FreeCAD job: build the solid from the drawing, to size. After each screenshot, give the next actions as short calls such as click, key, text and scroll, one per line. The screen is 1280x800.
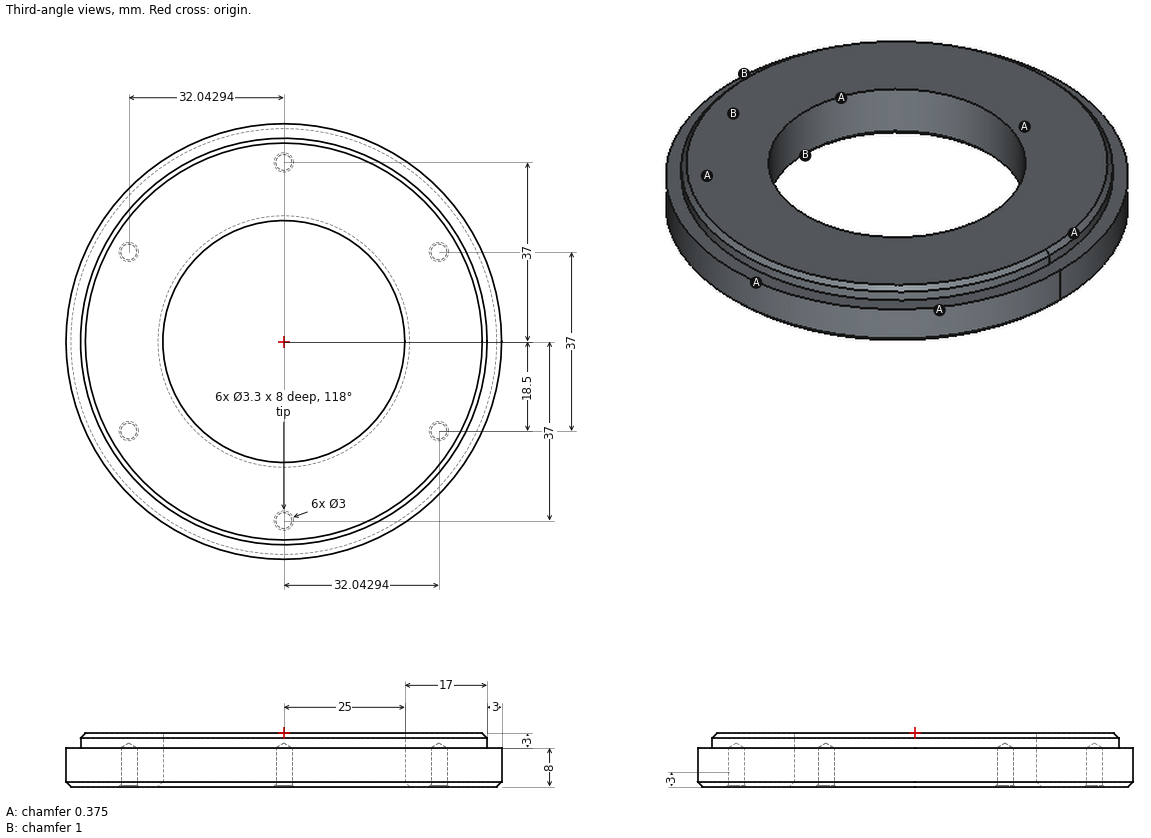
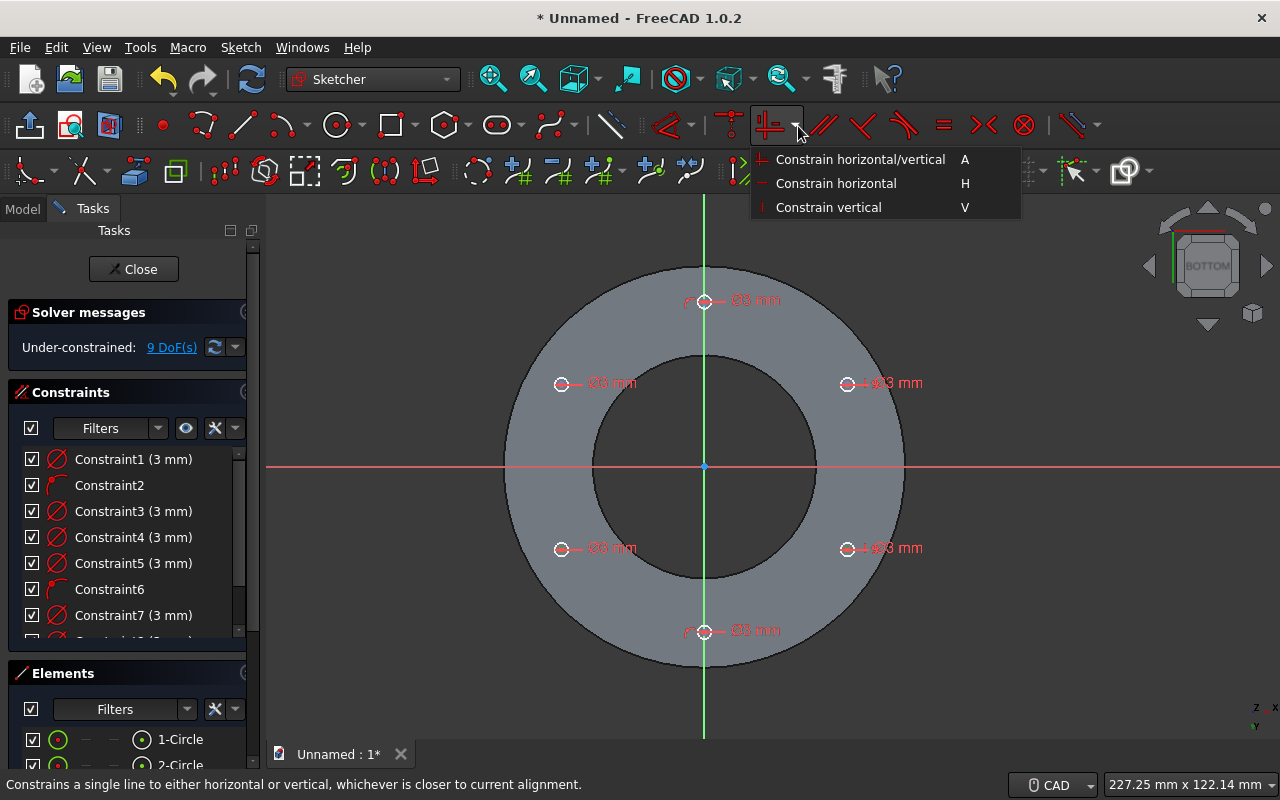
click(886, 183)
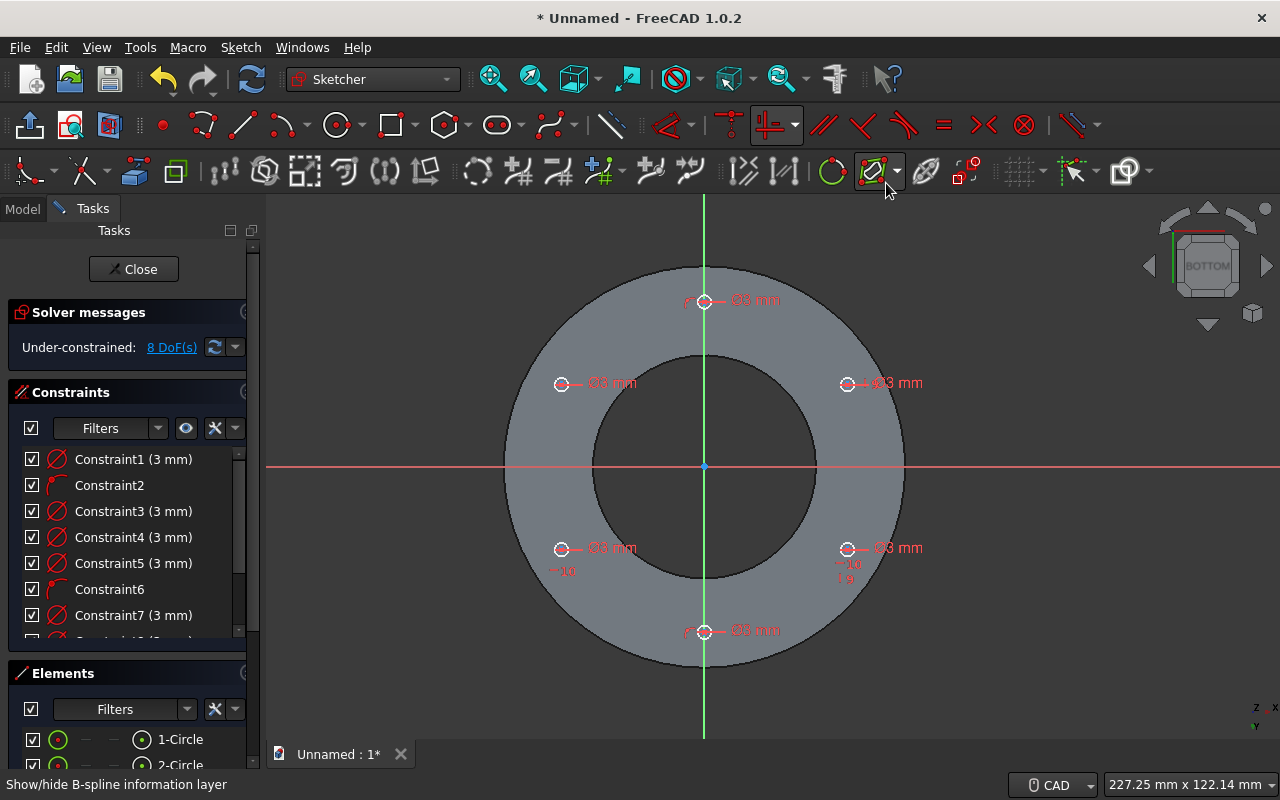
click(561, 550)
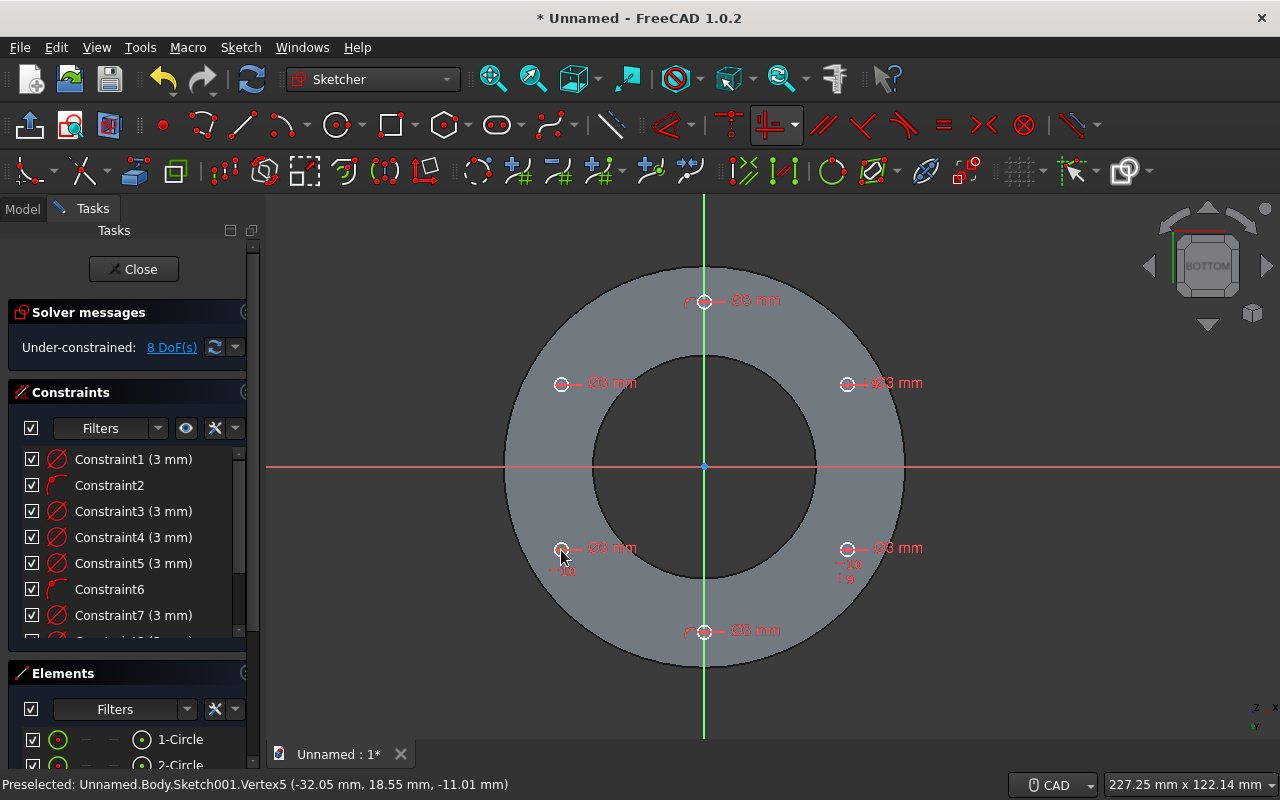
click(561, 385)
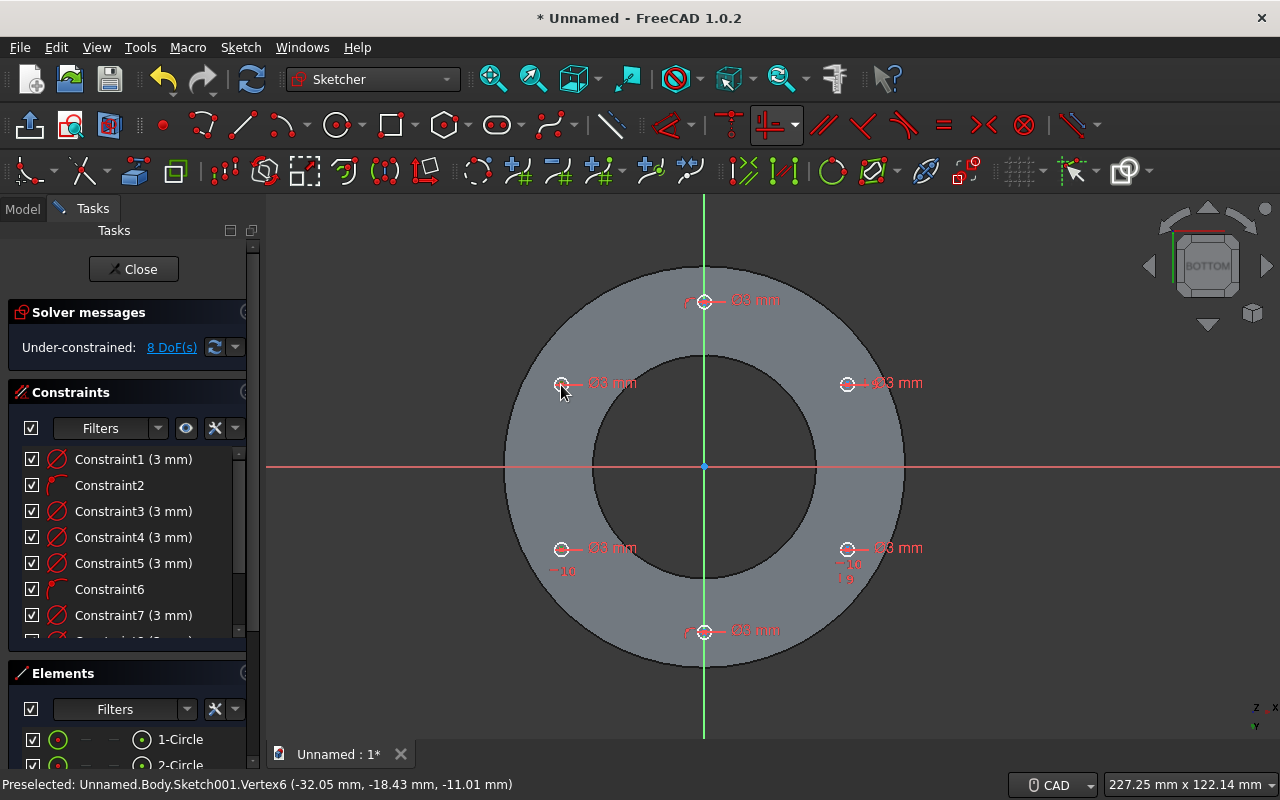
click(798, 126)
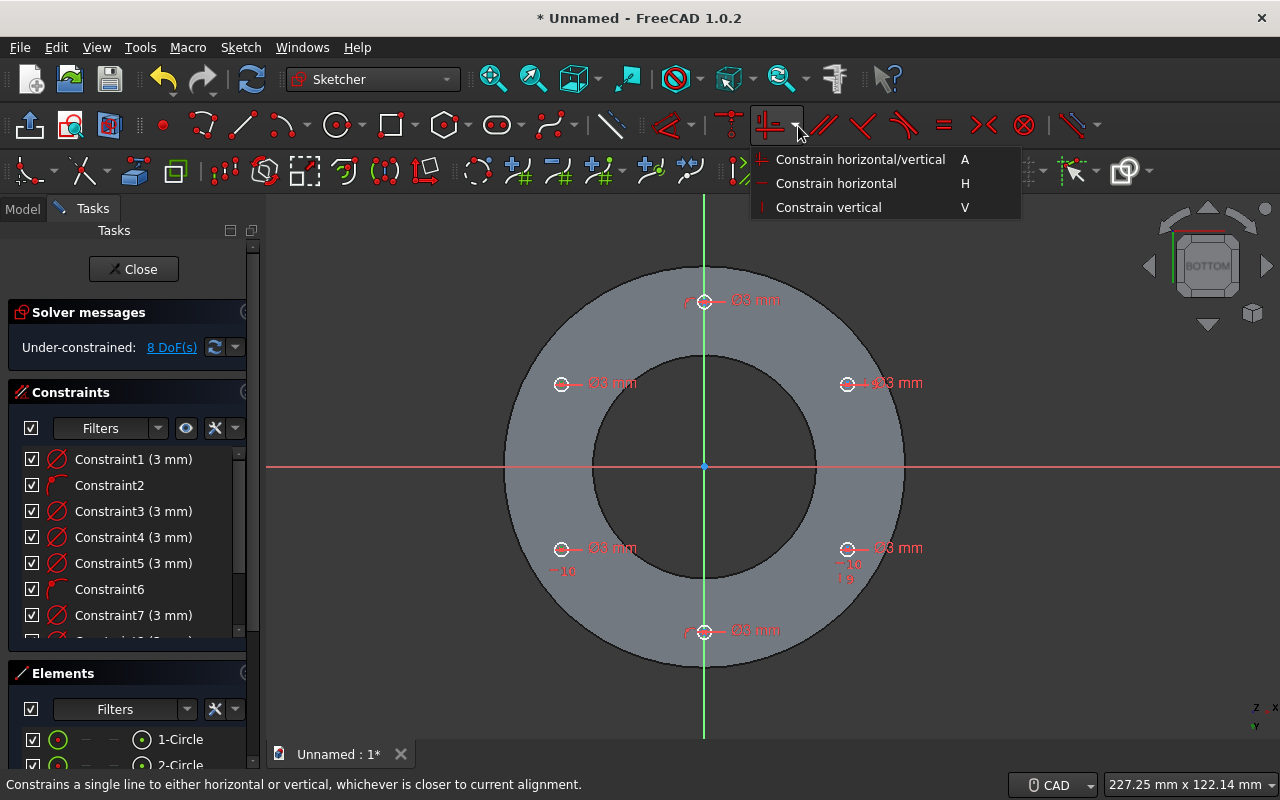
click(886, 207)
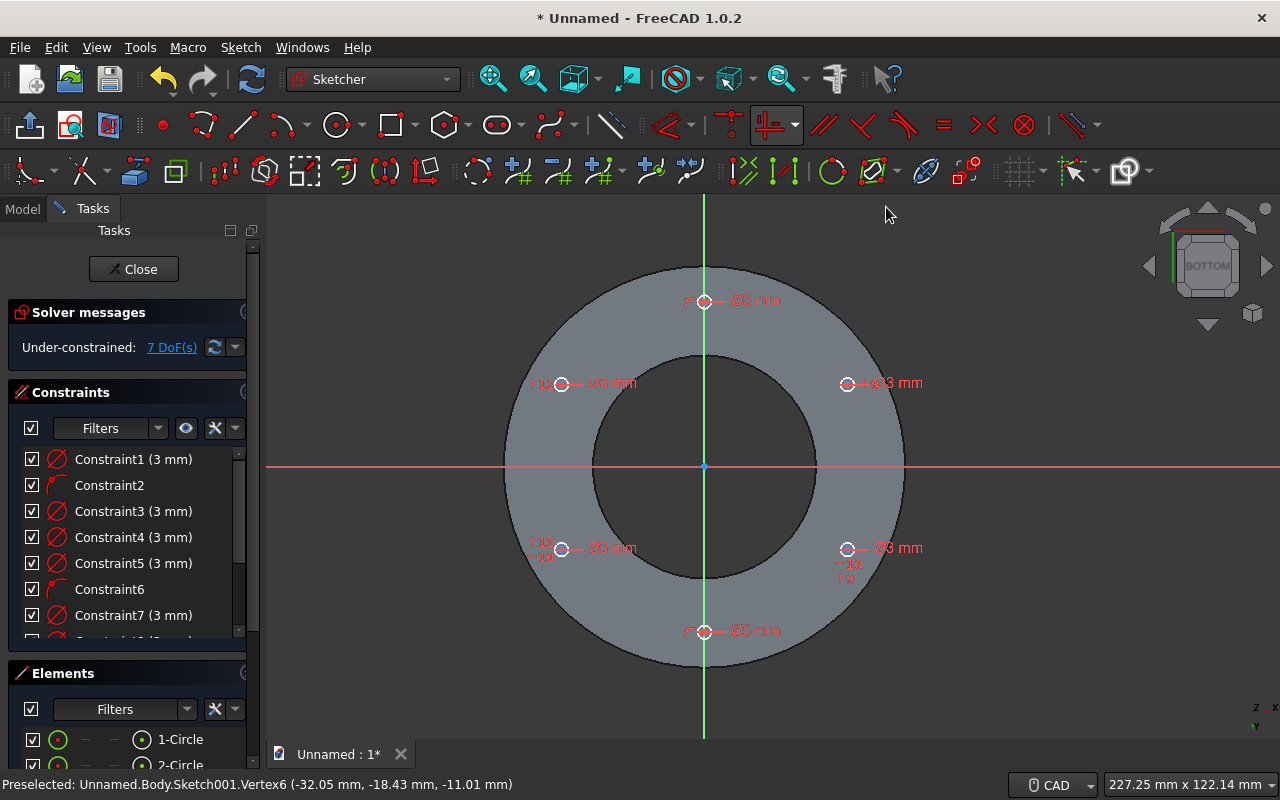
click(847, 385)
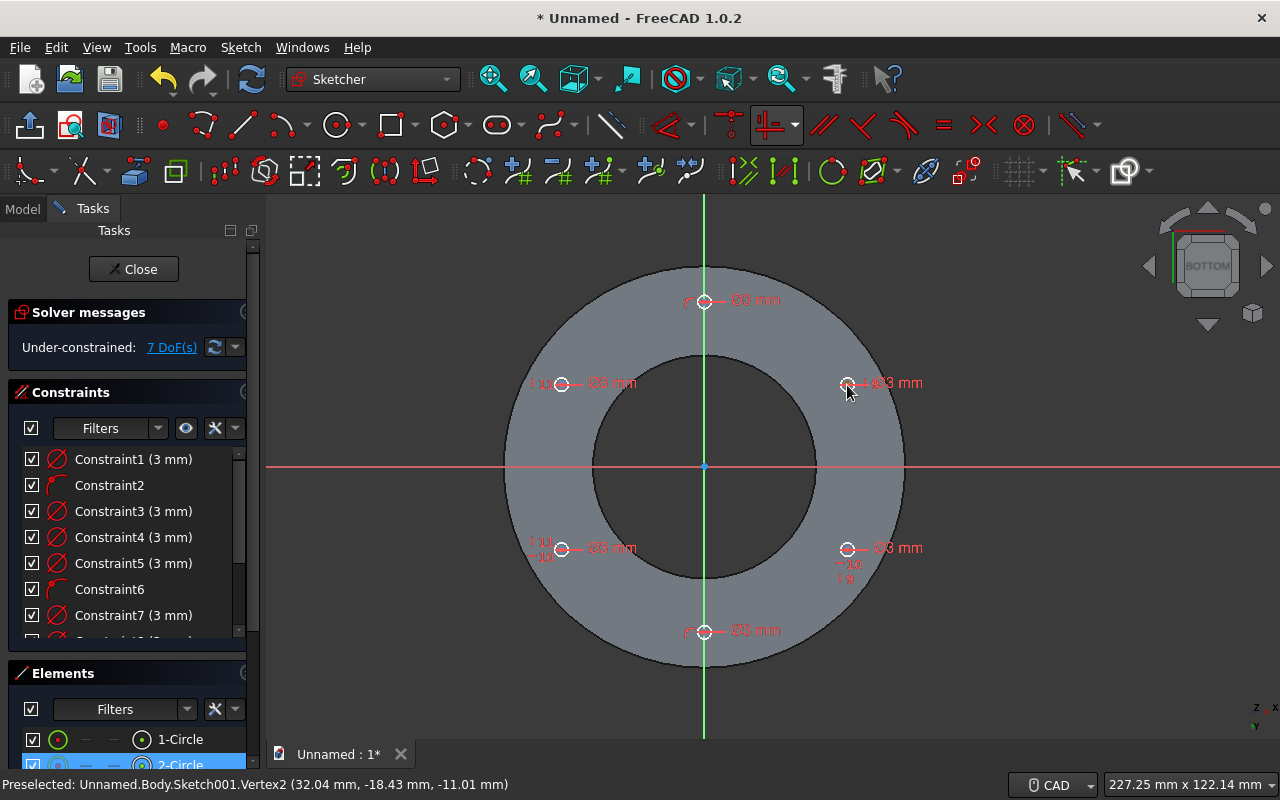
click(561, 385)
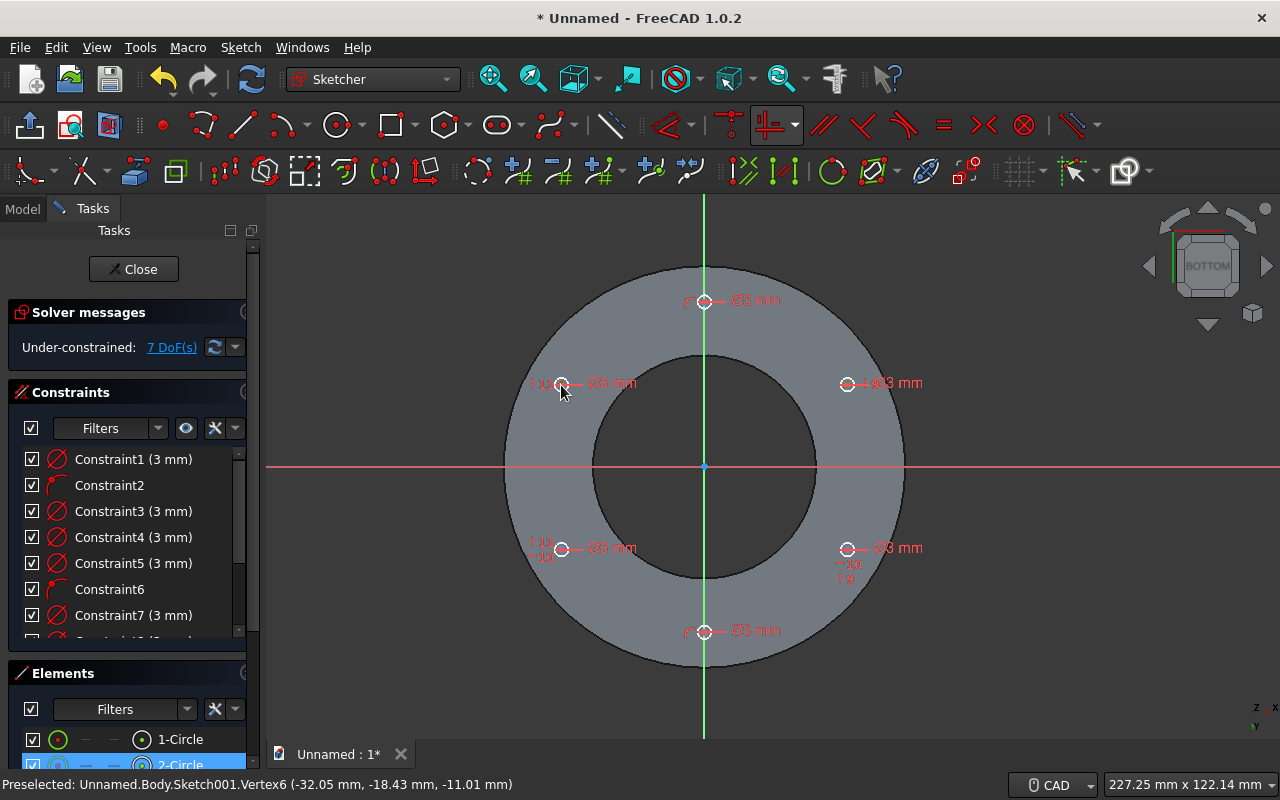
click(798, 126)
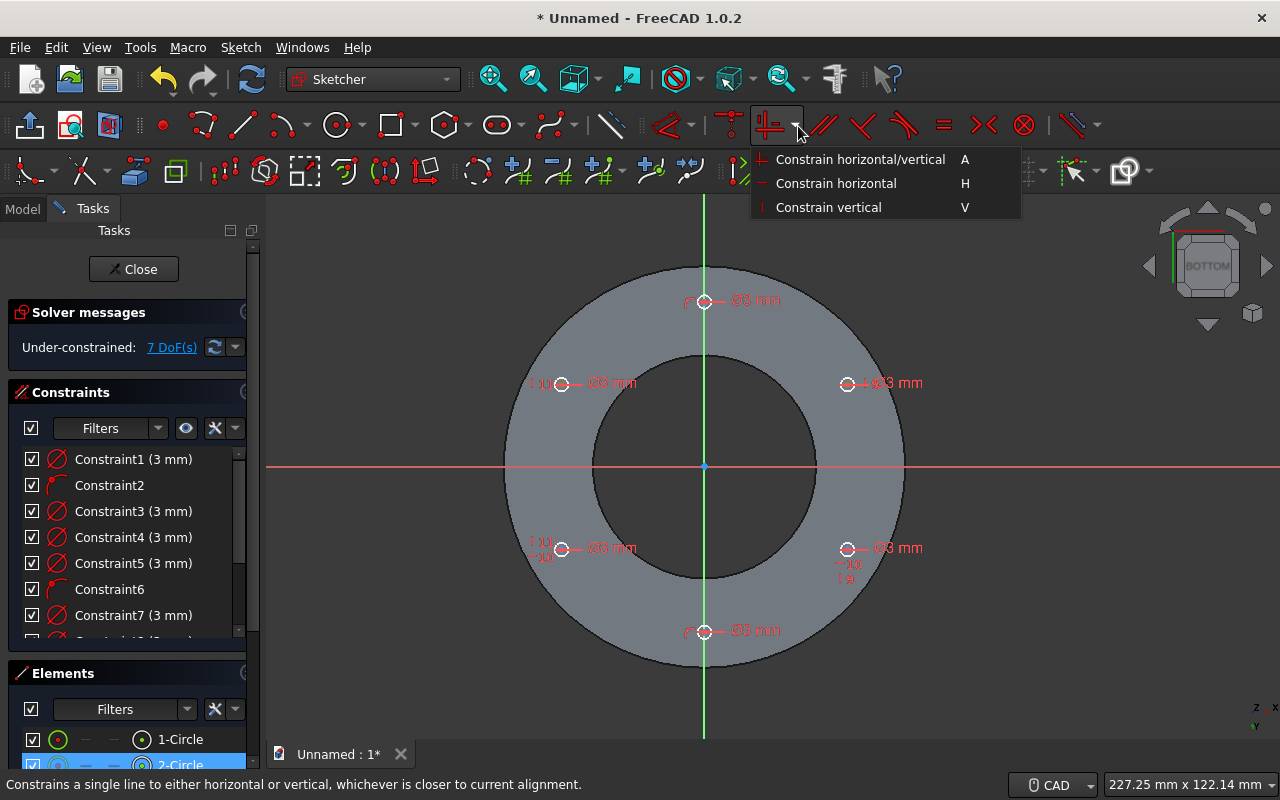
click(886, 183)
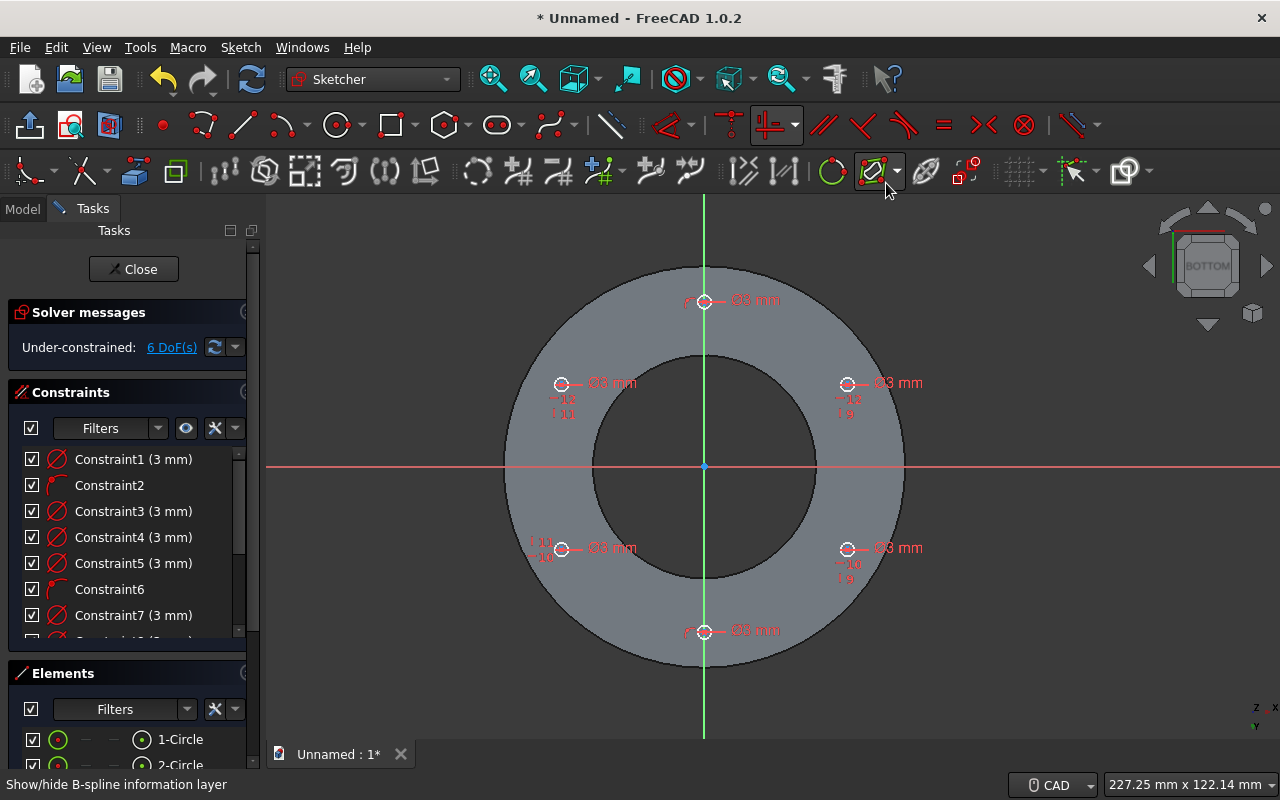
click(666, 126)